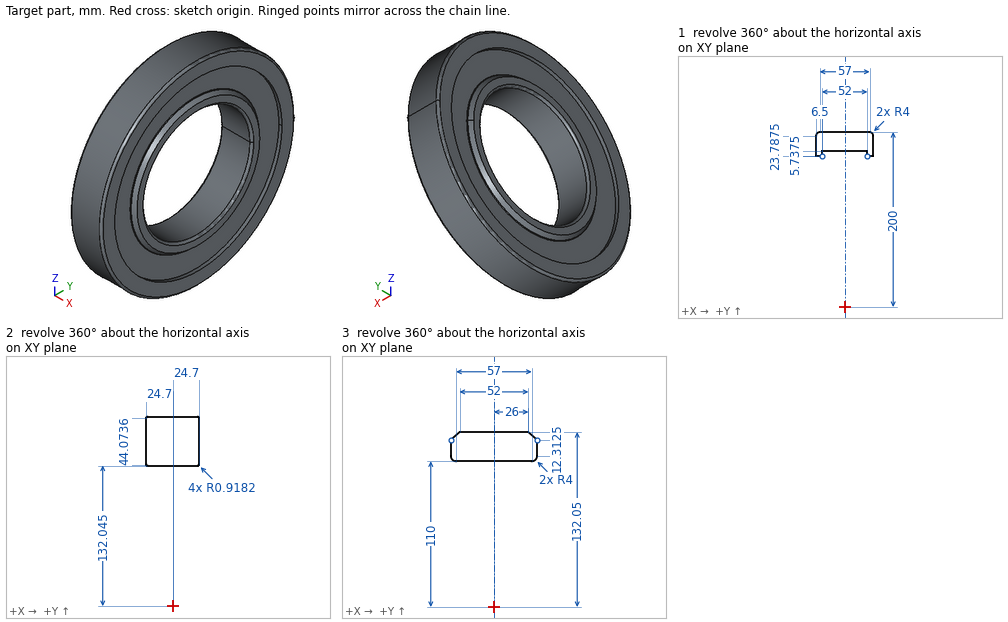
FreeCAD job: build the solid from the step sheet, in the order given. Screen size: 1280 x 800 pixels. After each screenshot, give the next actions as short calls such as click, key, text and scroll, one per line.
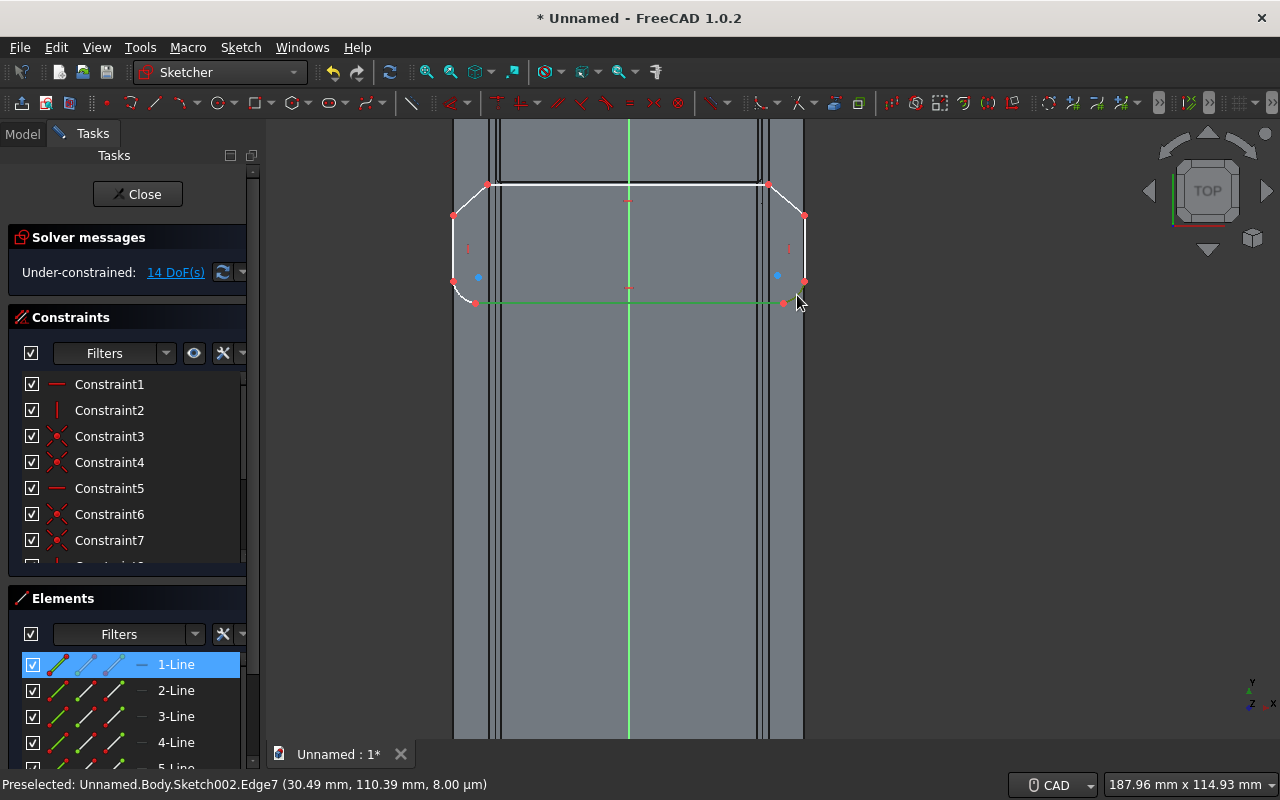
click(606, 104)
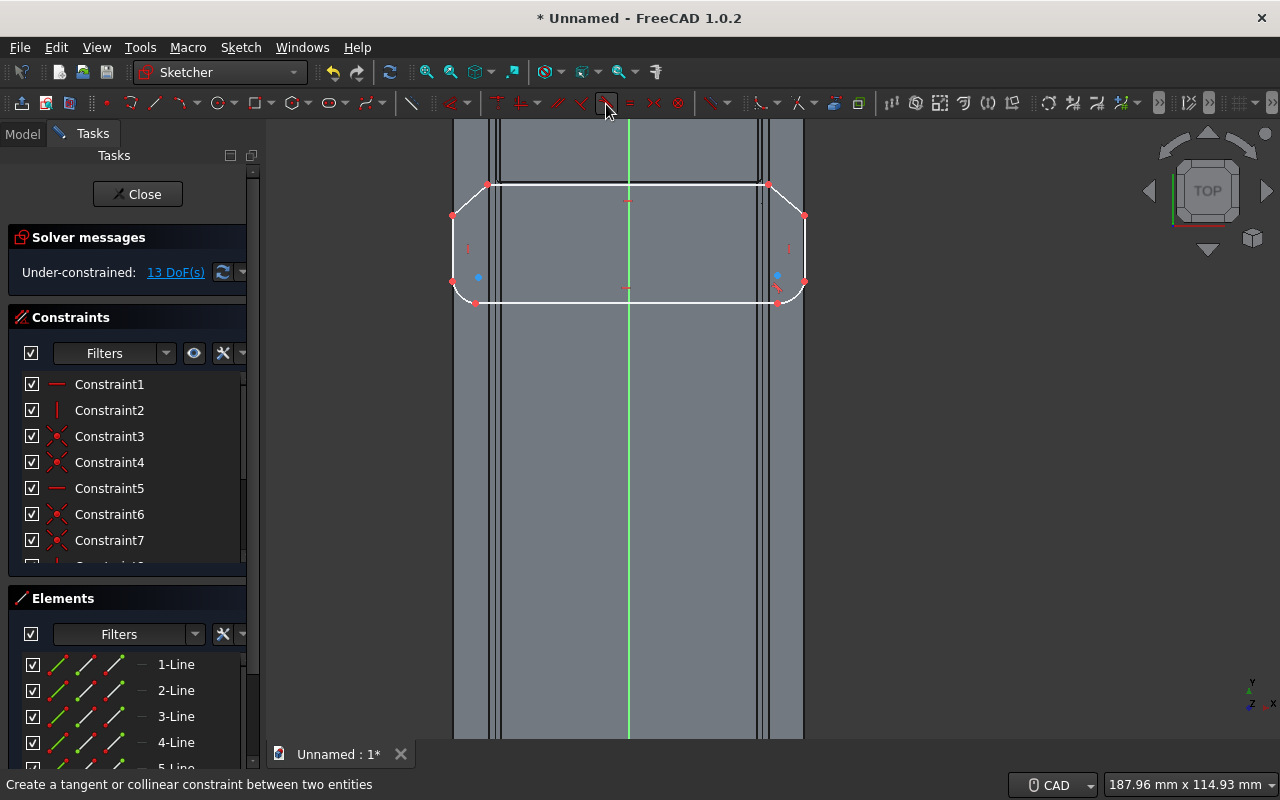
click(566, 303)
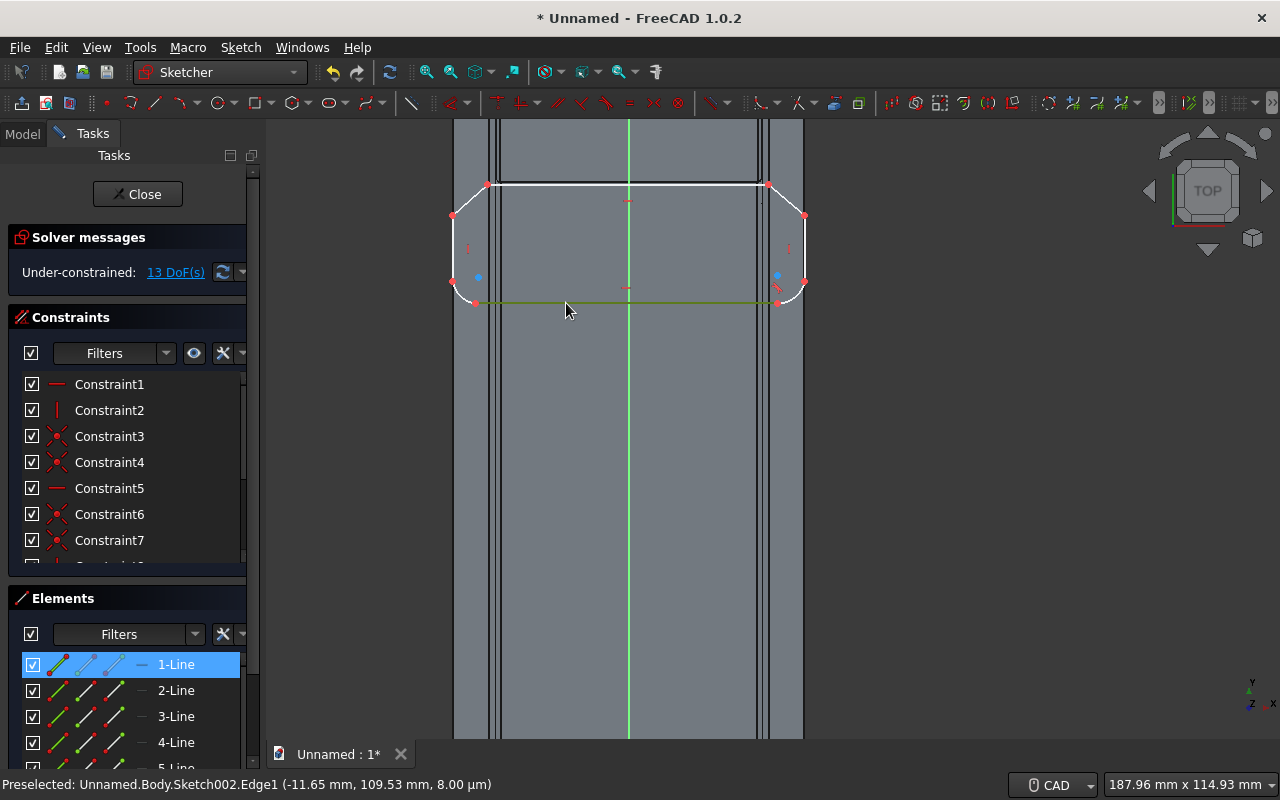
scroll(456, 291, up, 2)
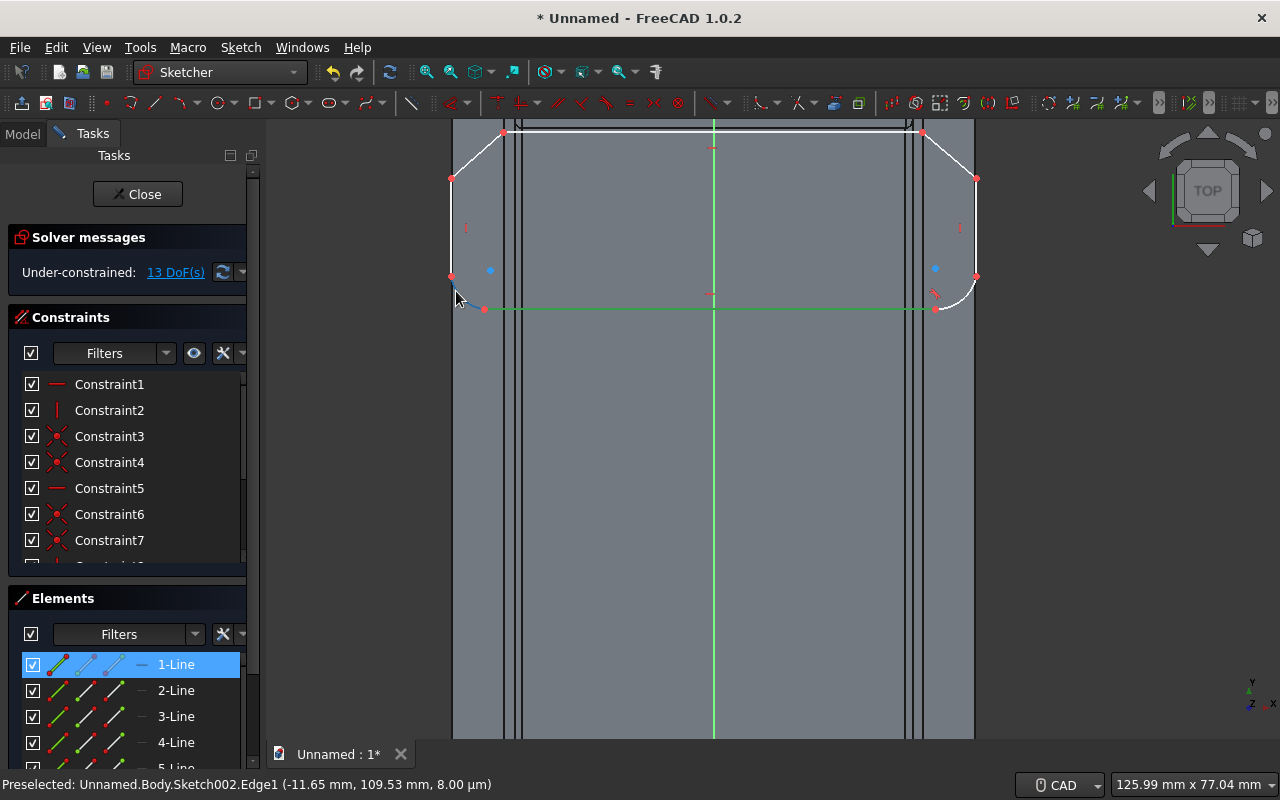
click(456, 290)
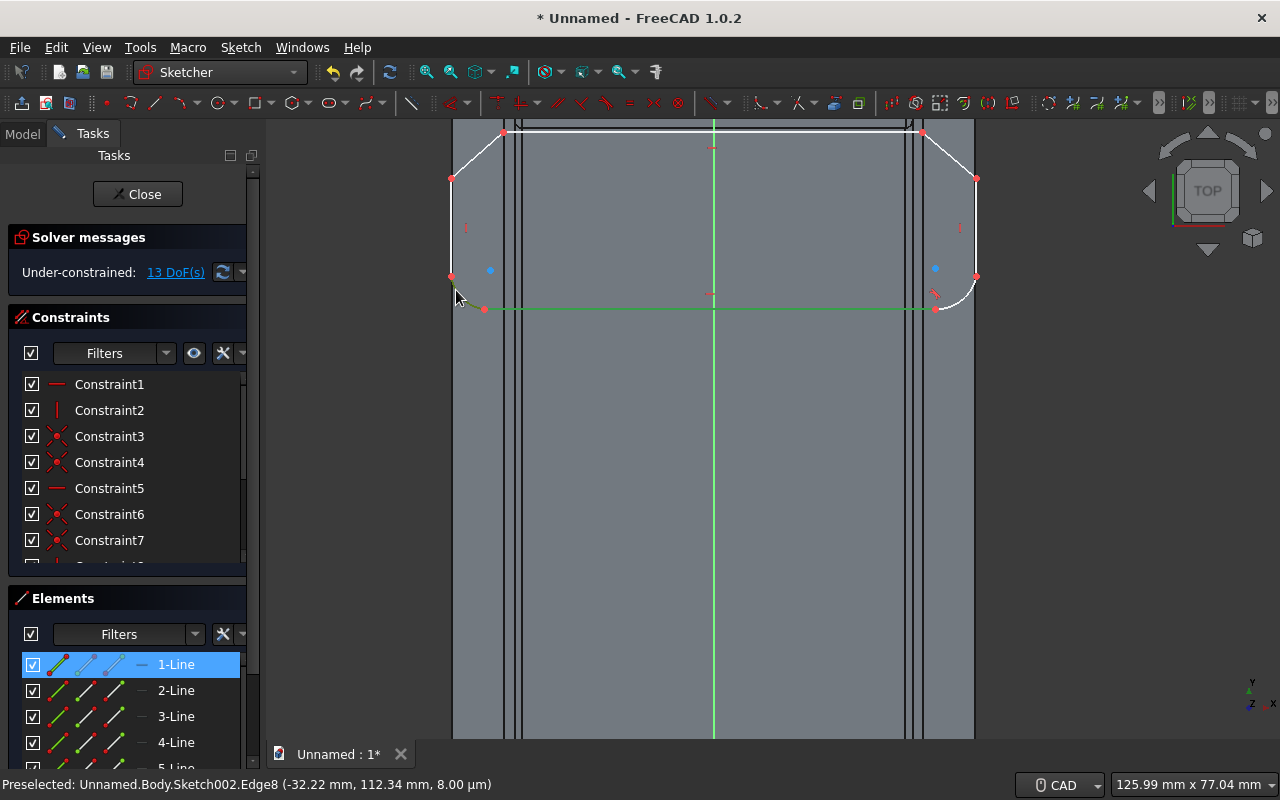
click(606, 104)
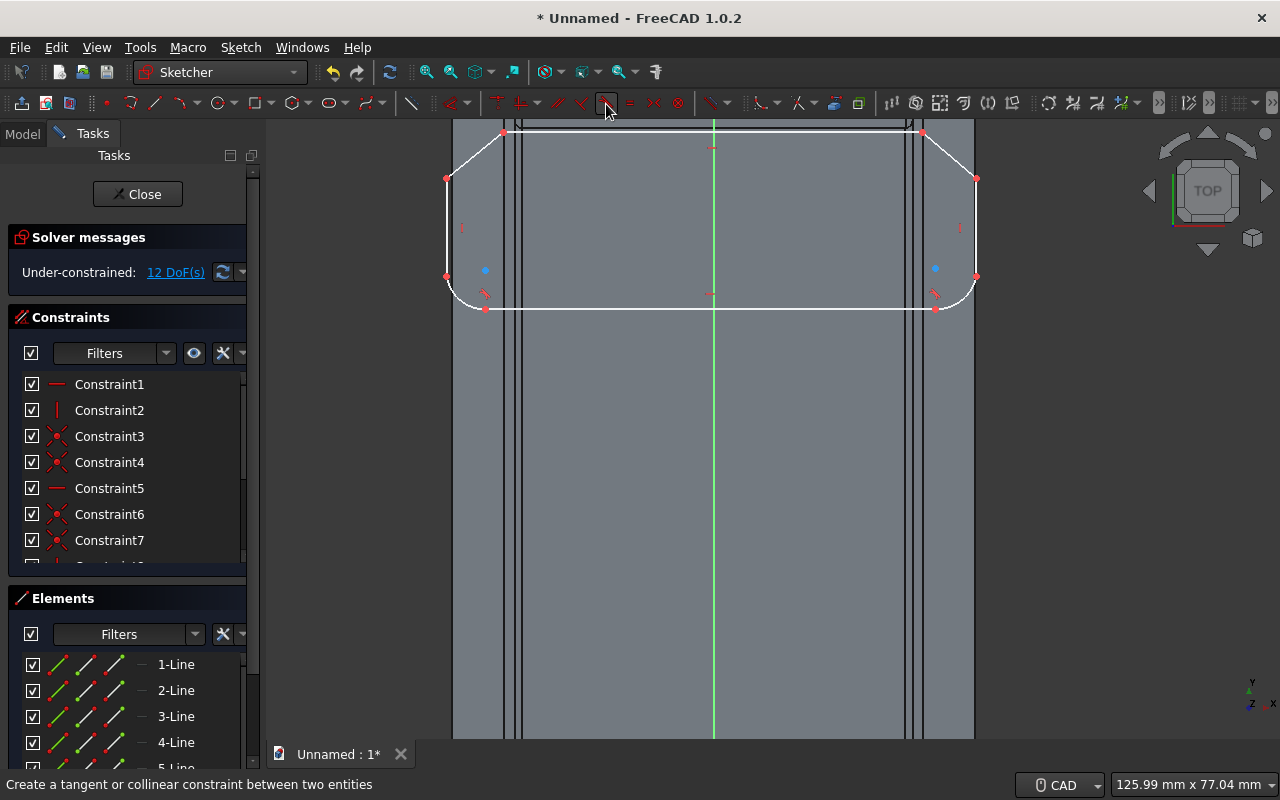
click(976, 247)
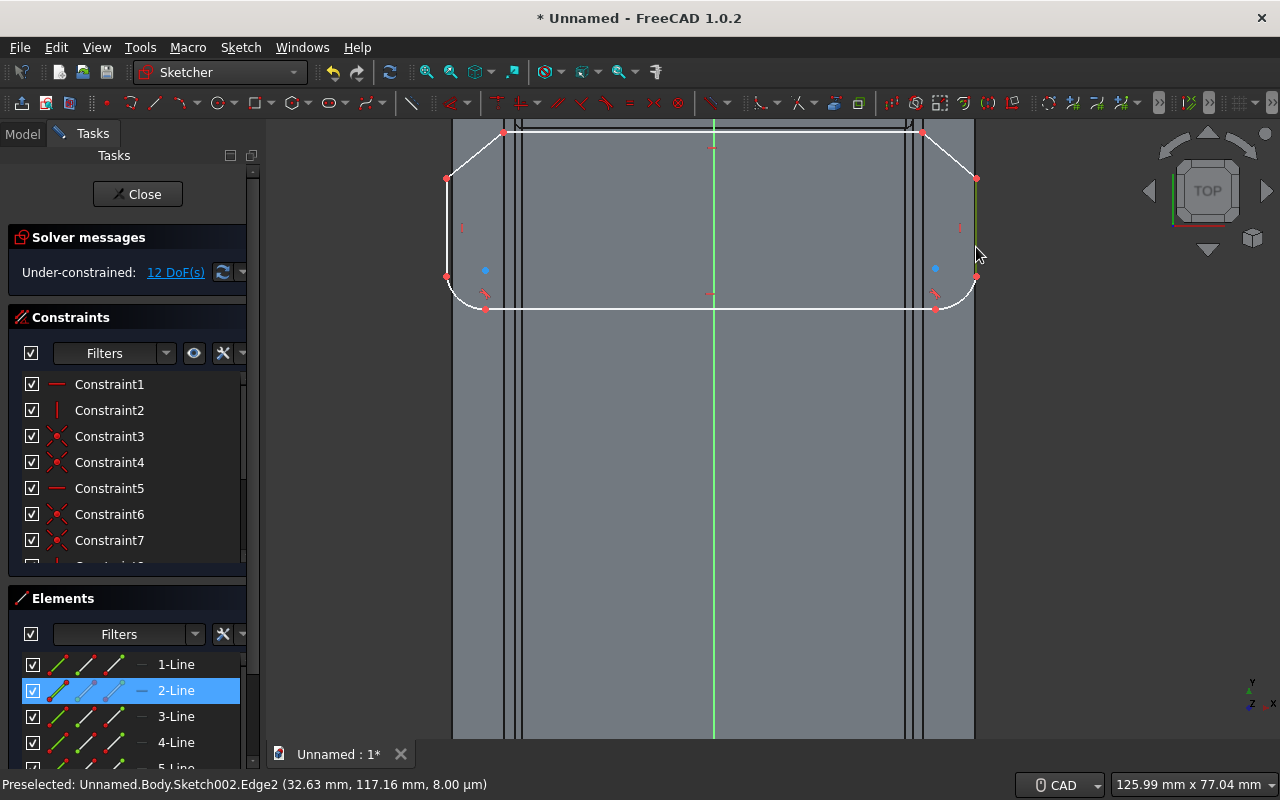
click(952, 306)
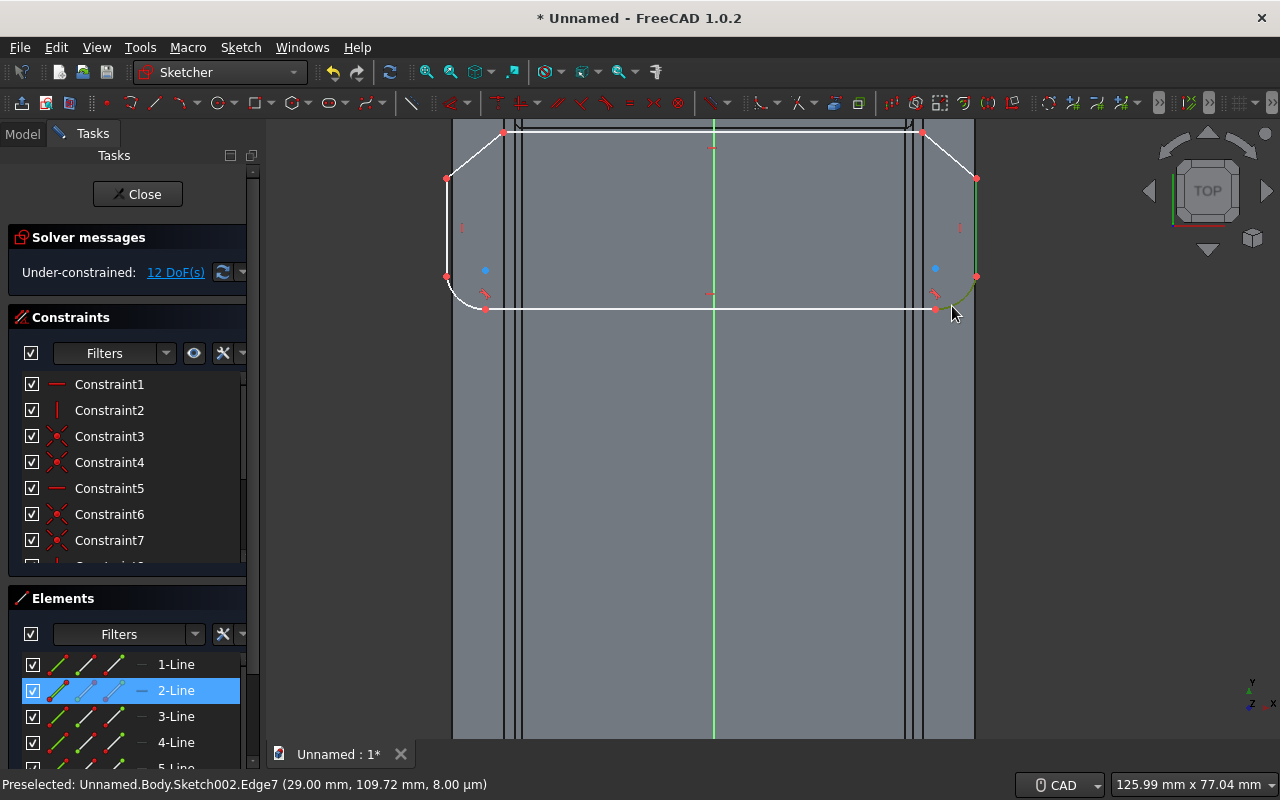
click(606, 104)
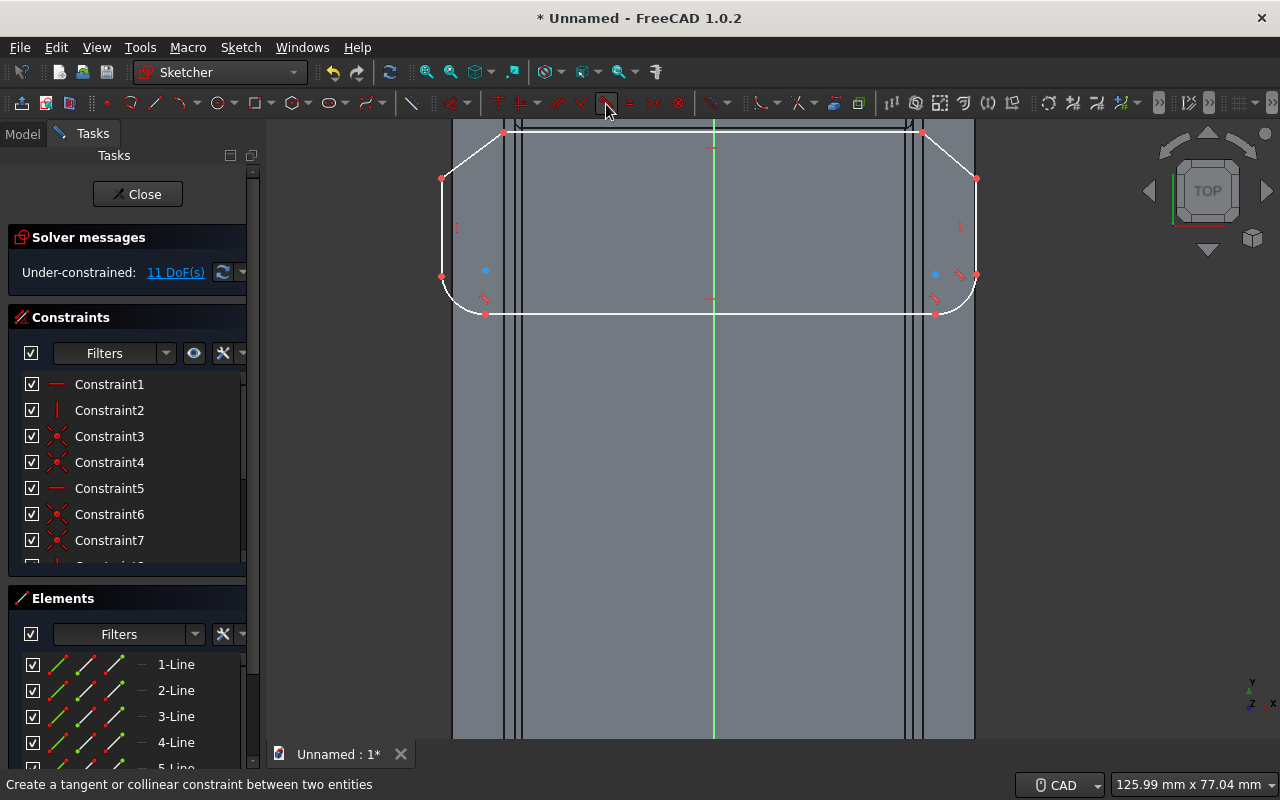
click(442, 208)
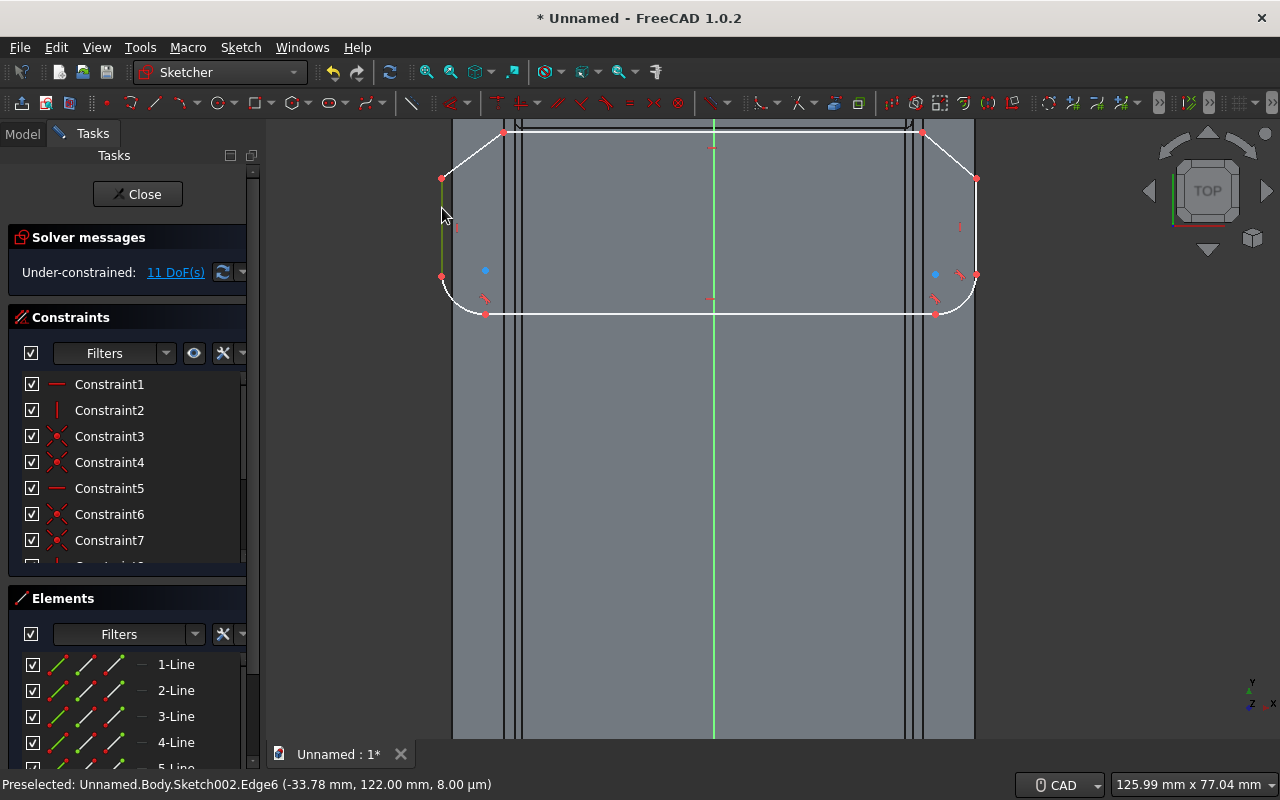
click(448, 294)